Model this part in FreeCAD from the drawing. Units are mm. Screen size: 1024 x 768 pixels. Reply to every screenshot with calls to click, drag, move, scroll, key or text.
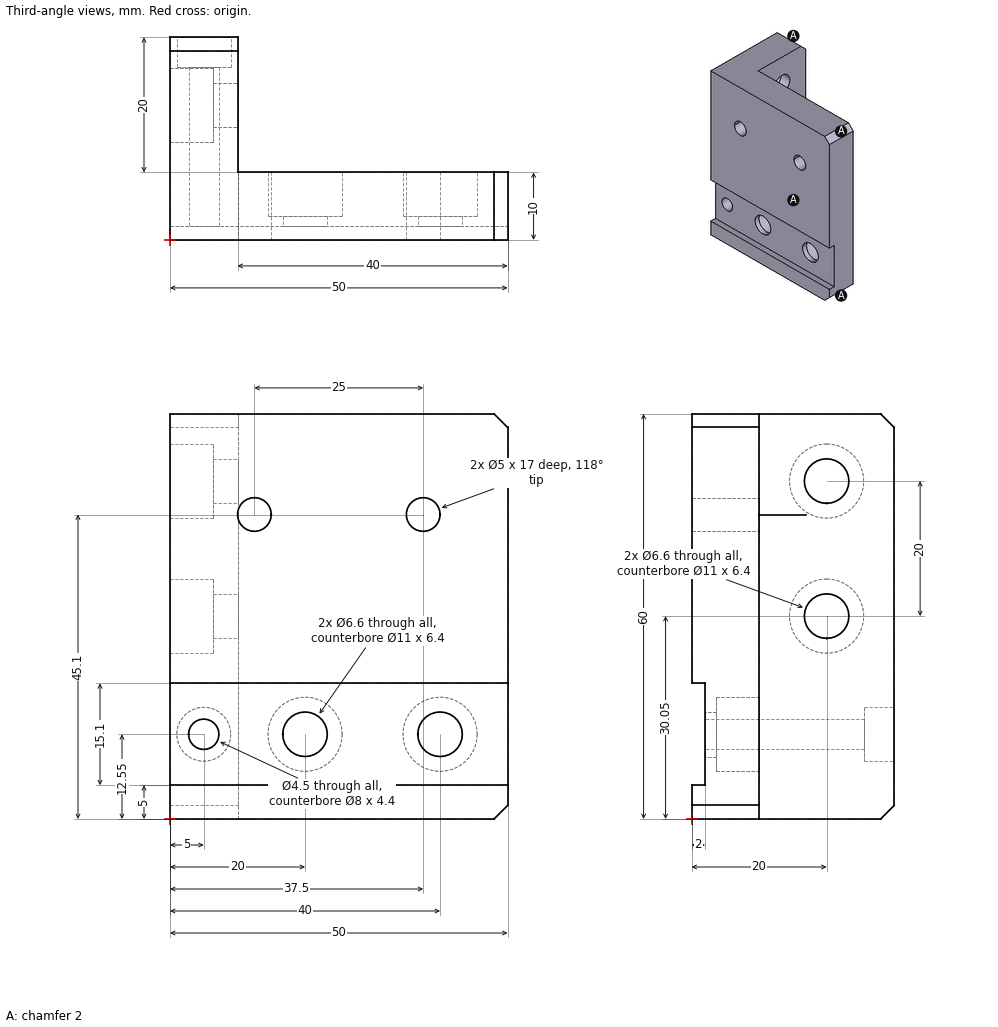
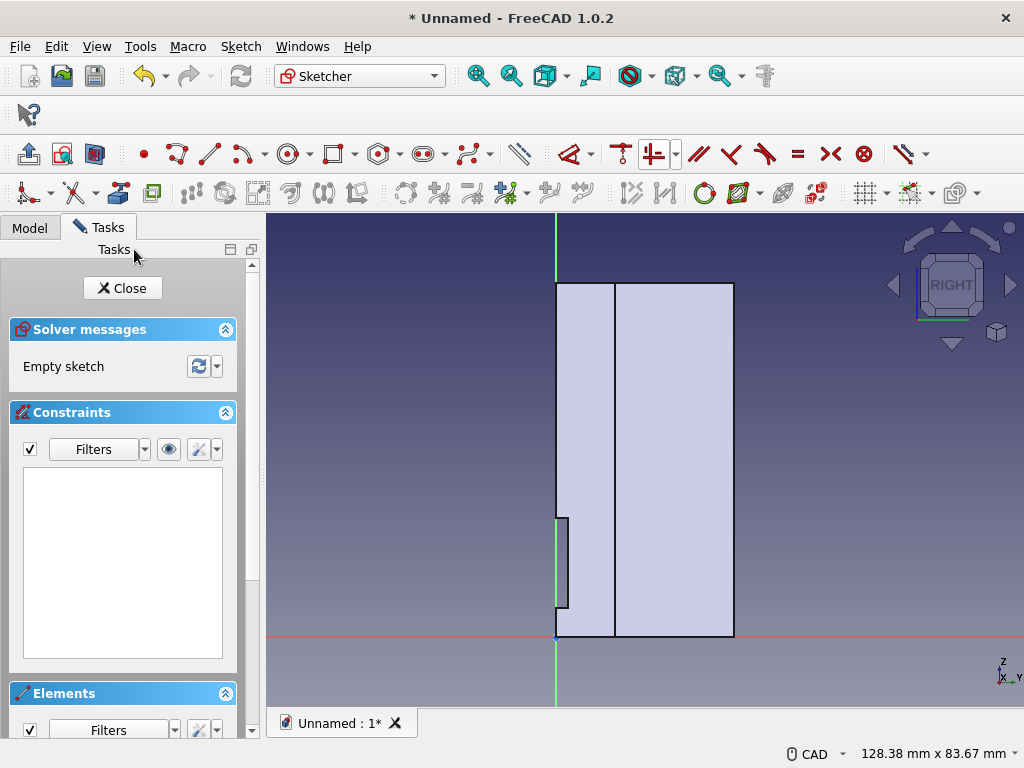
click(95, 154)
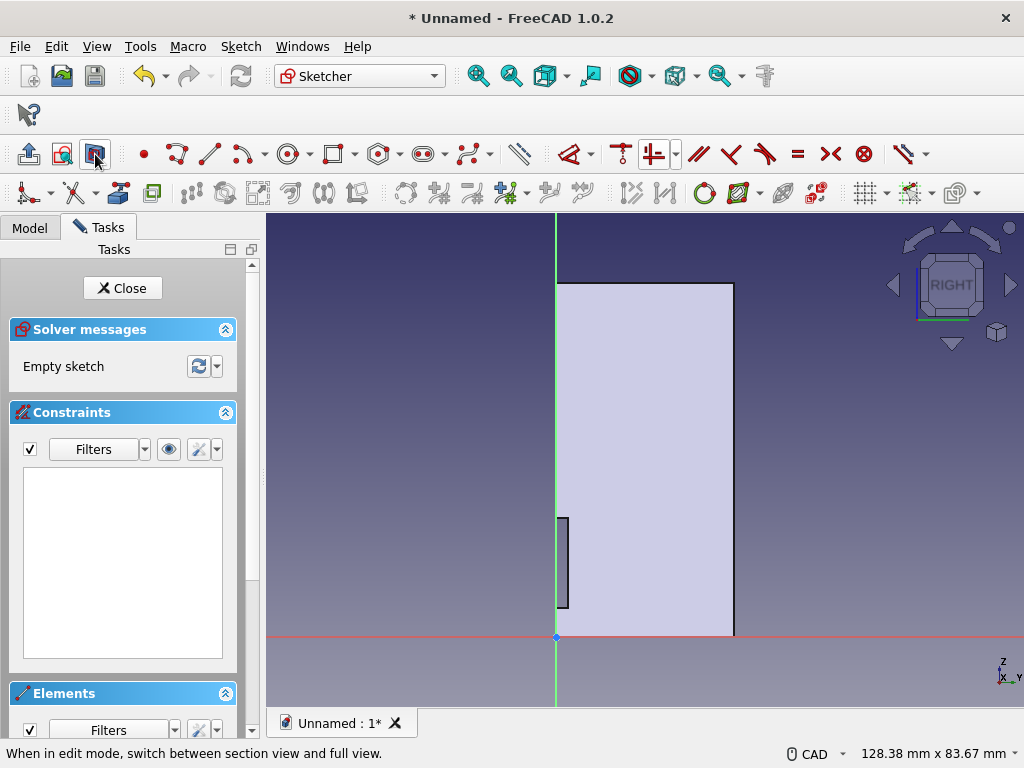
click(288, 154)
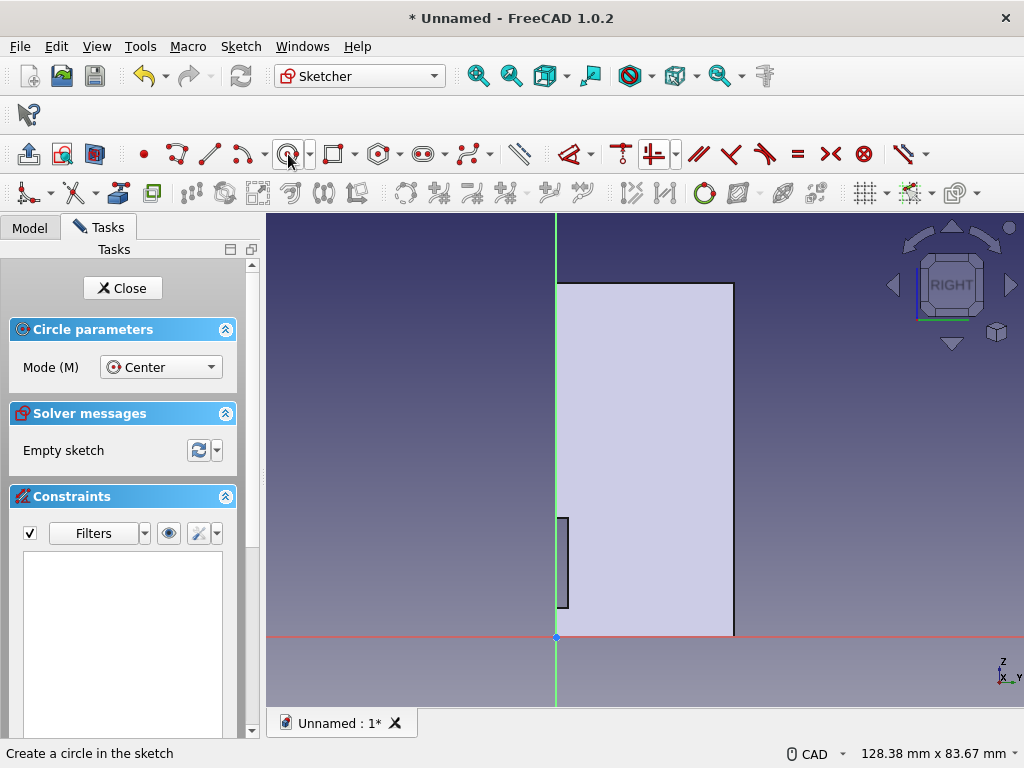
click(675, 460)
click(688, 446)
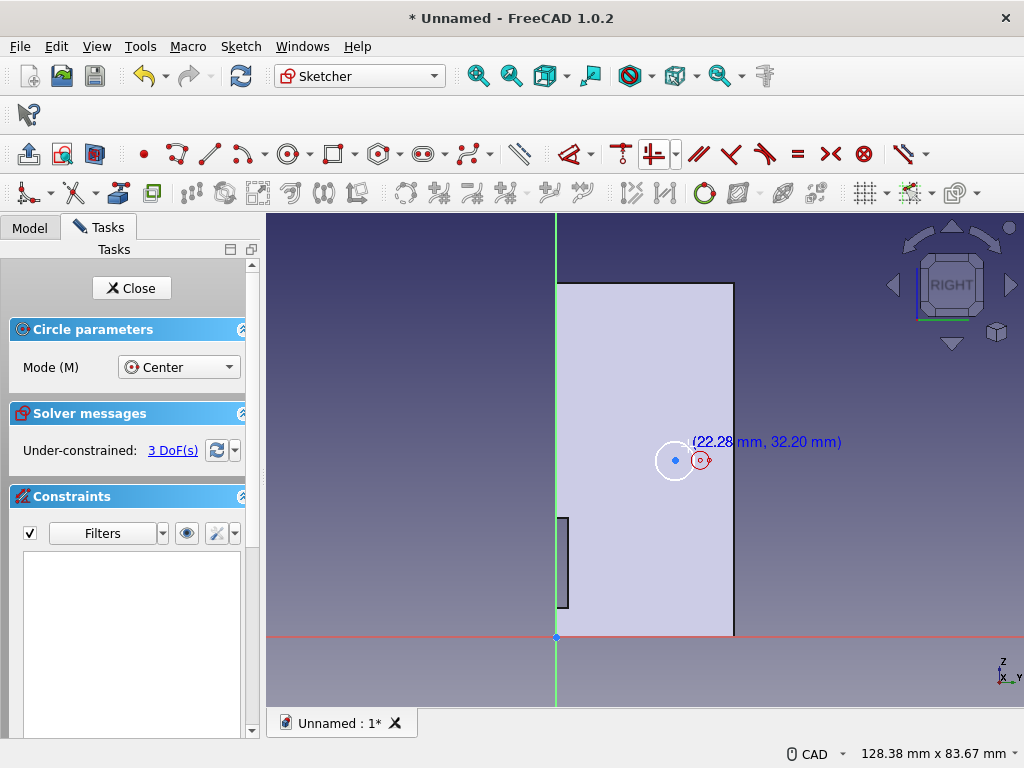
click(675, 342)
click(688, 328)
key(Escape)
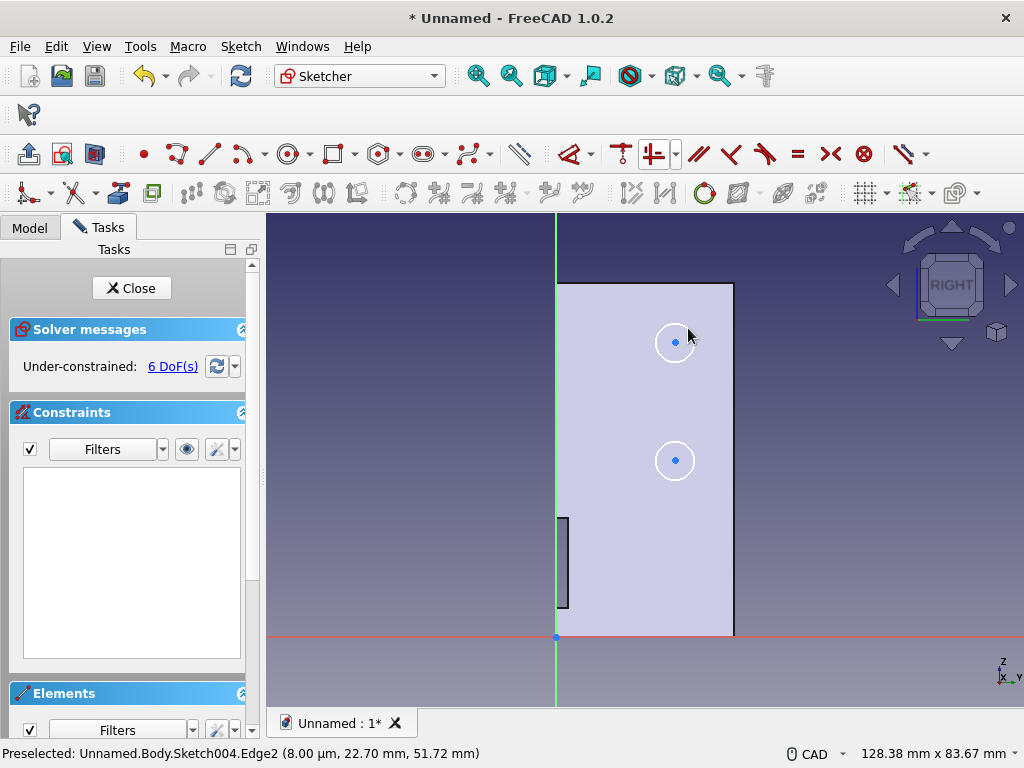
click(688, 447)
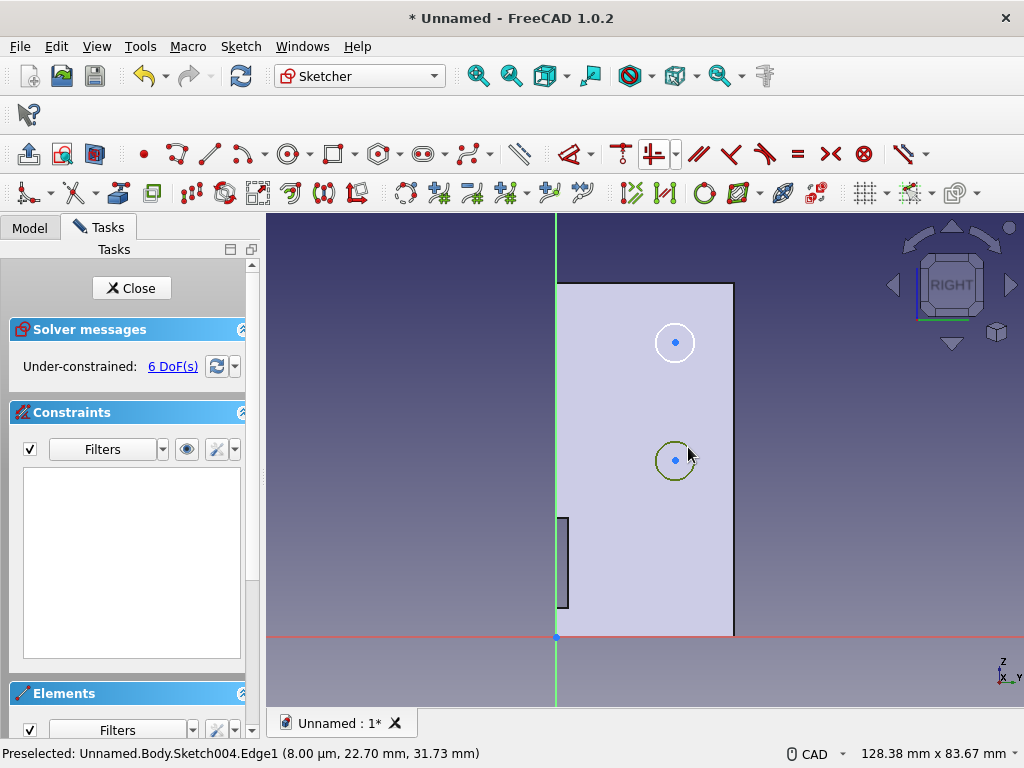
click(688, 329)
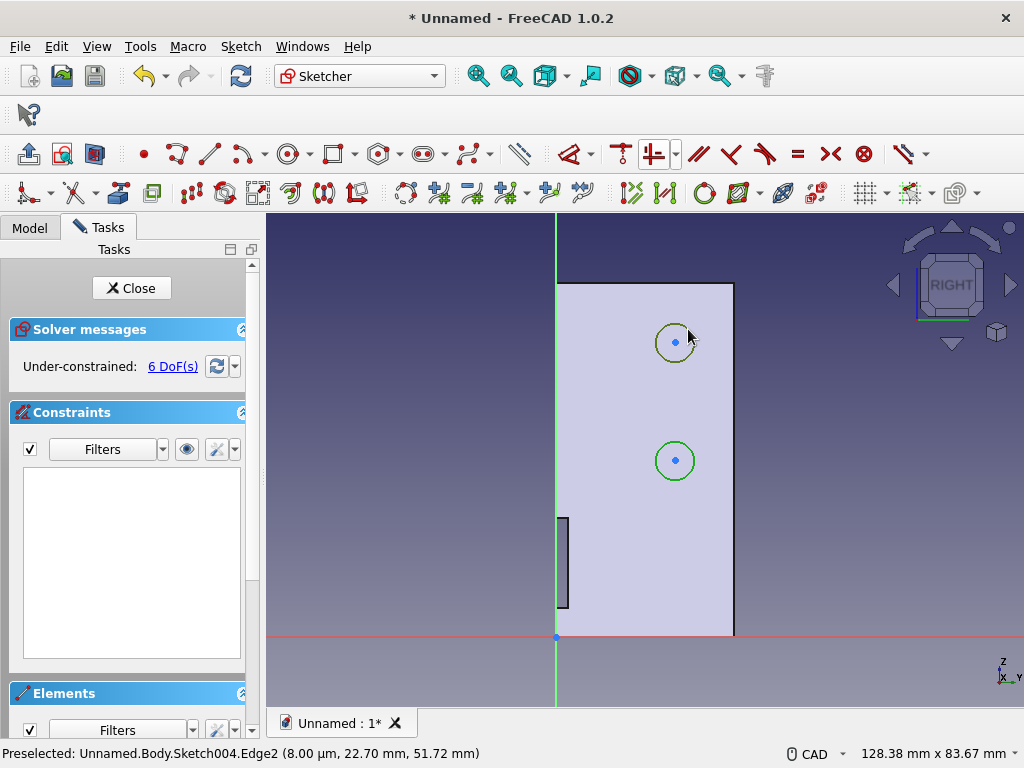
click(798, 154)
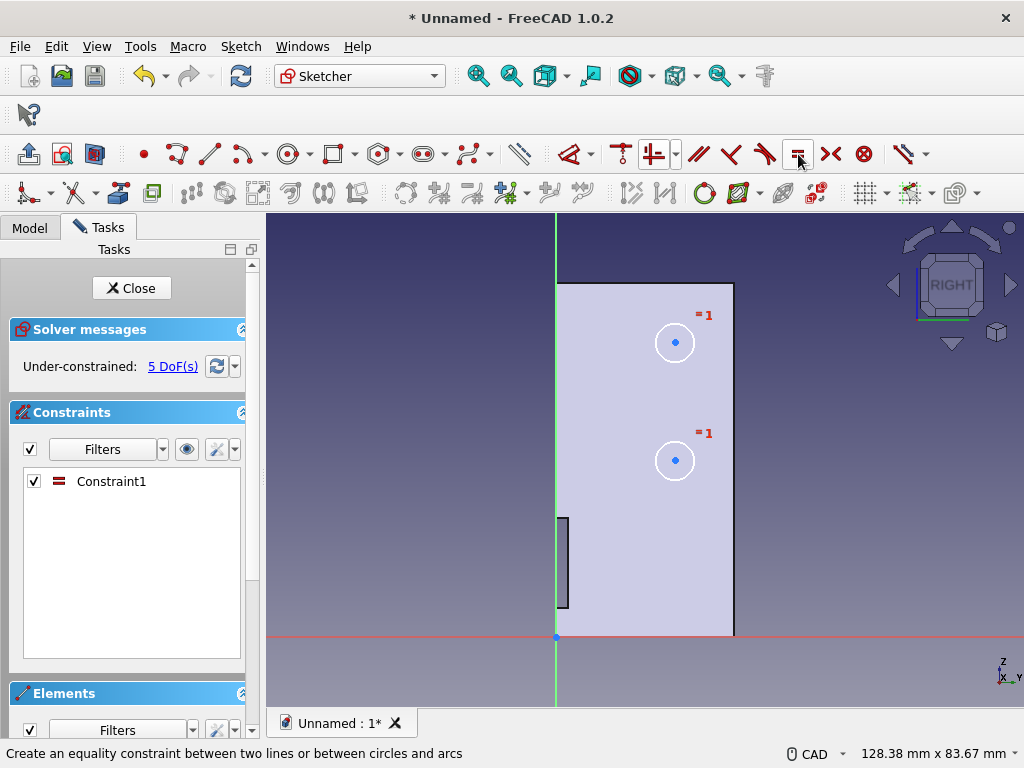
click(568, 154)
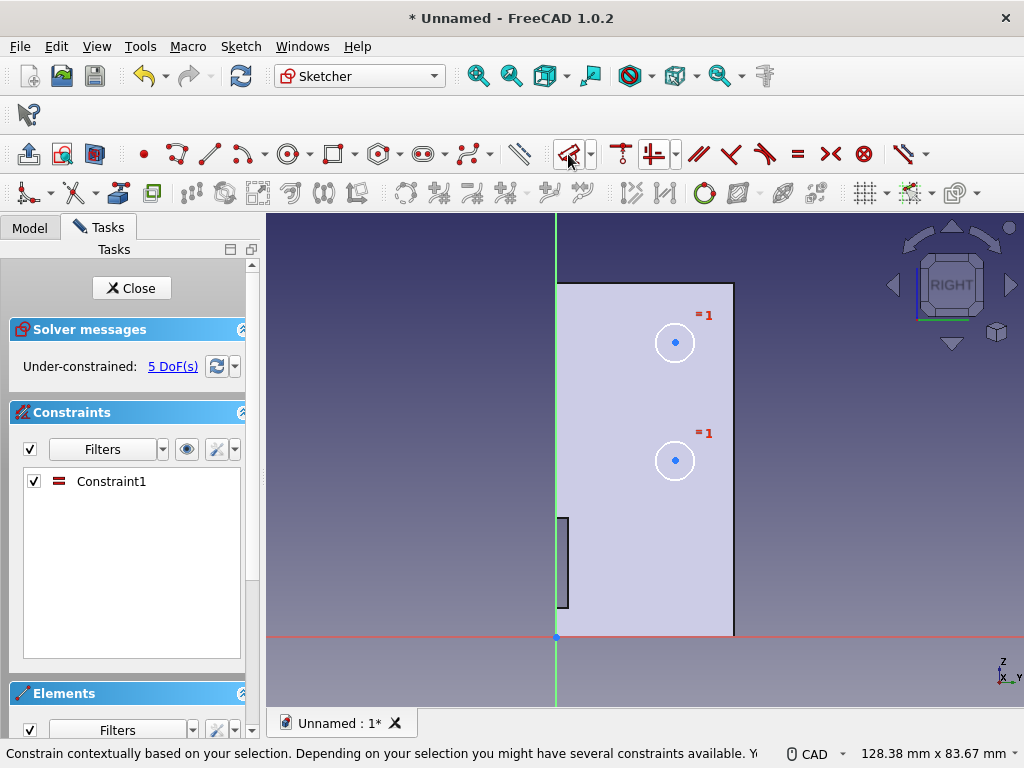
click(688, 447)
click(710, 424)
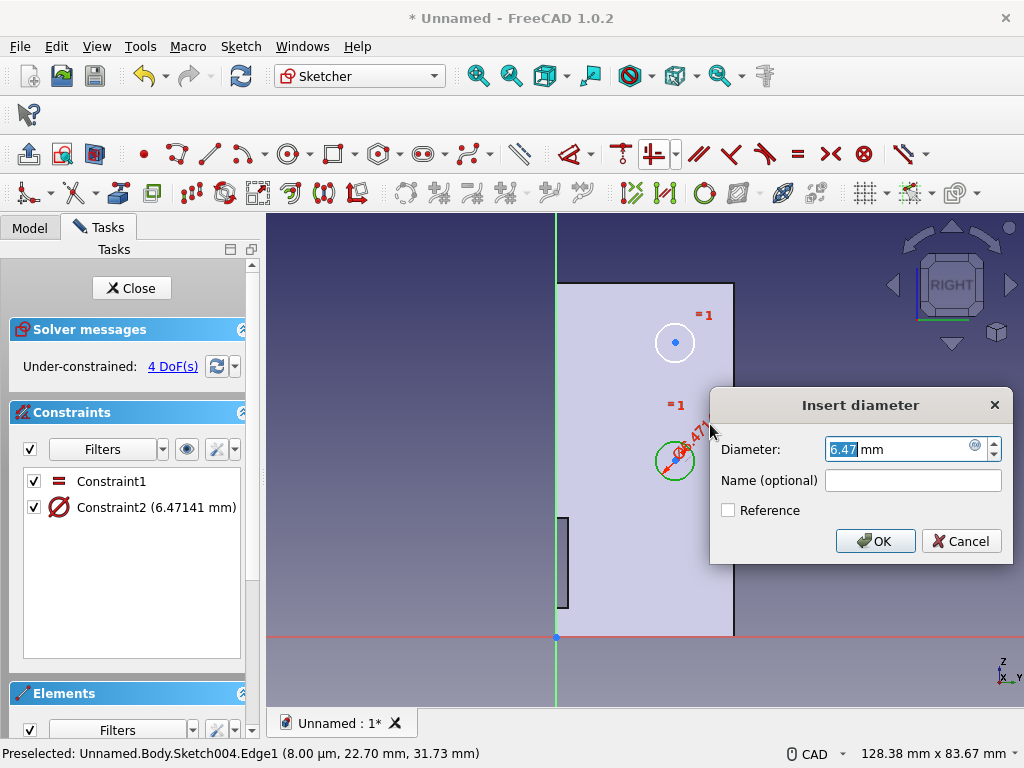
text(6.6)
key(Return)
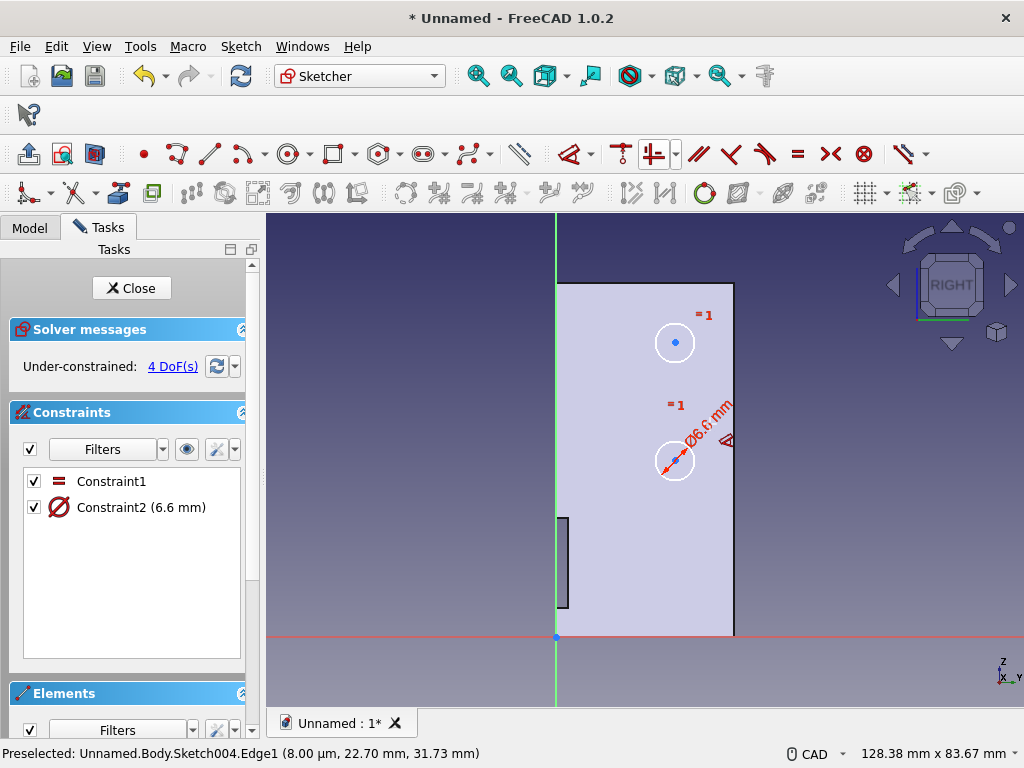
click(675, 461)
click(616, 671)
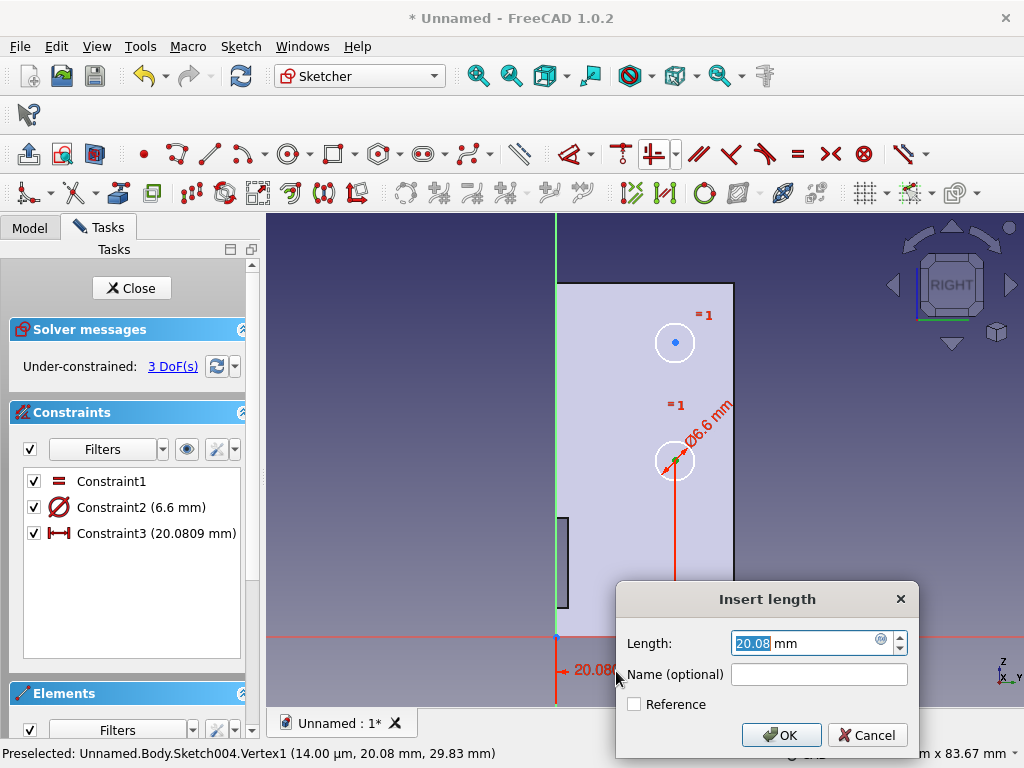
text(20)
key(Return)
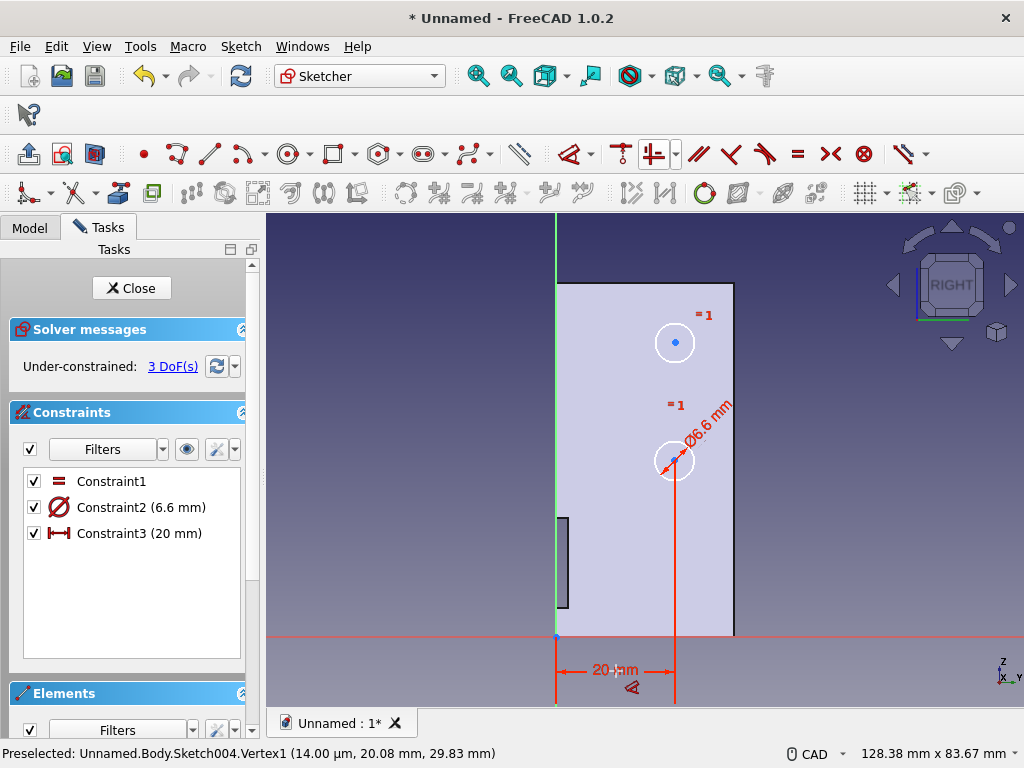
click(675, 343)
click(616, 309)